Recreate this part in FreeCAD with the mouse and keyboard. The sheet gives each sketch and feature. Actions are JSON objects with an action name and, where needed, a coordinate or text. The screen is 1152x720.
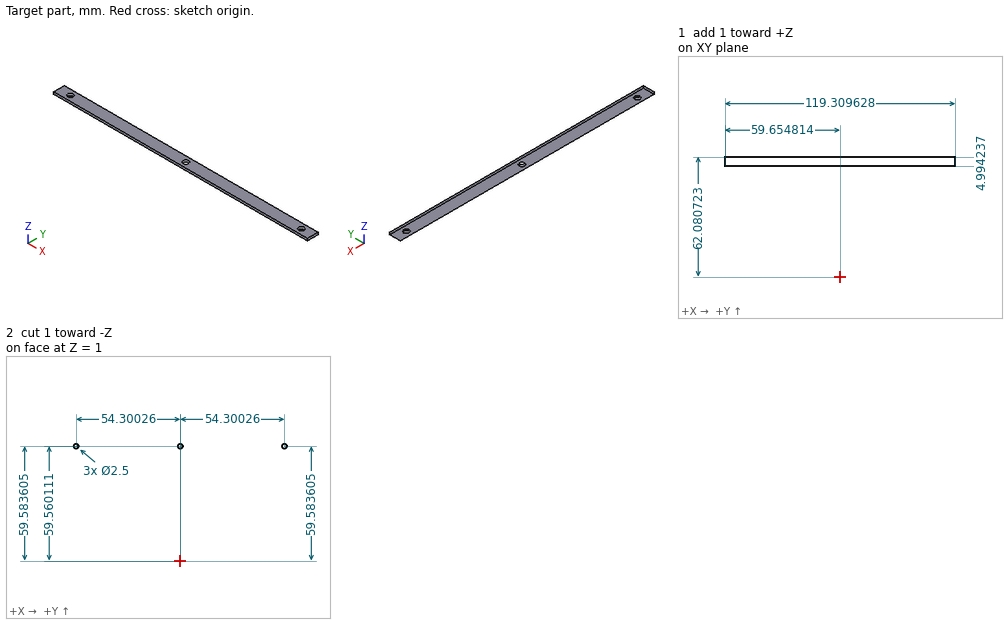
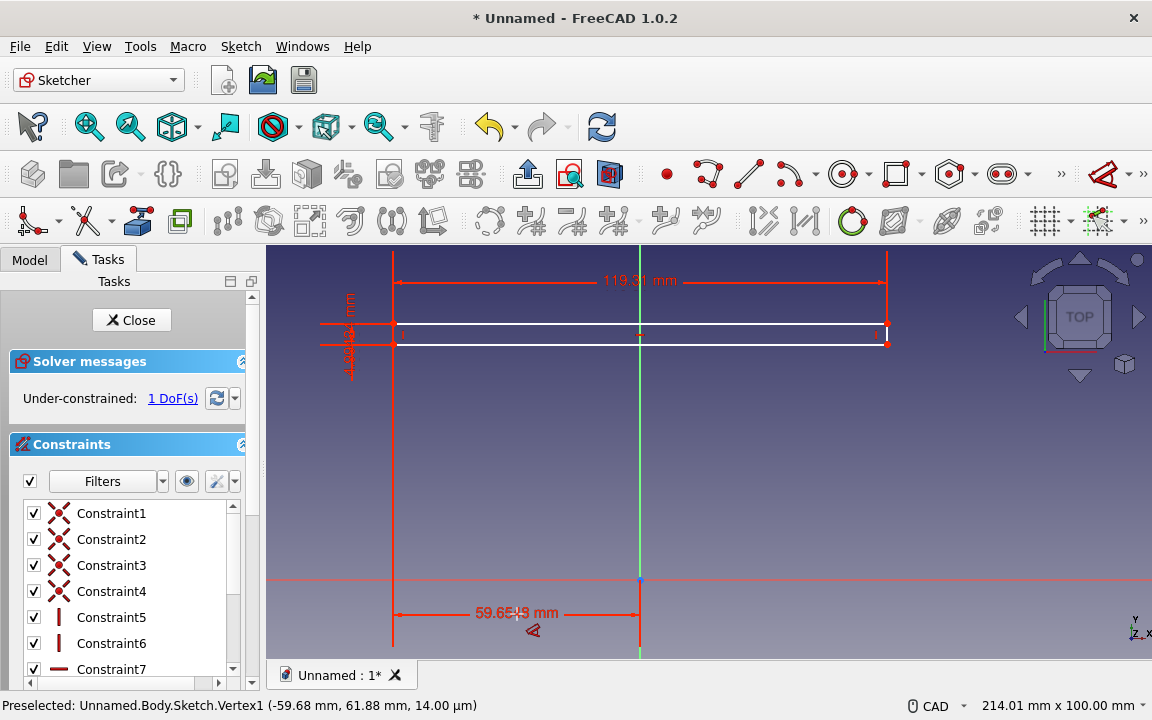
{"action": "left_click", "coordinate": [393, 324]}
{"action": "left_click", "coordinate": [359, 452]}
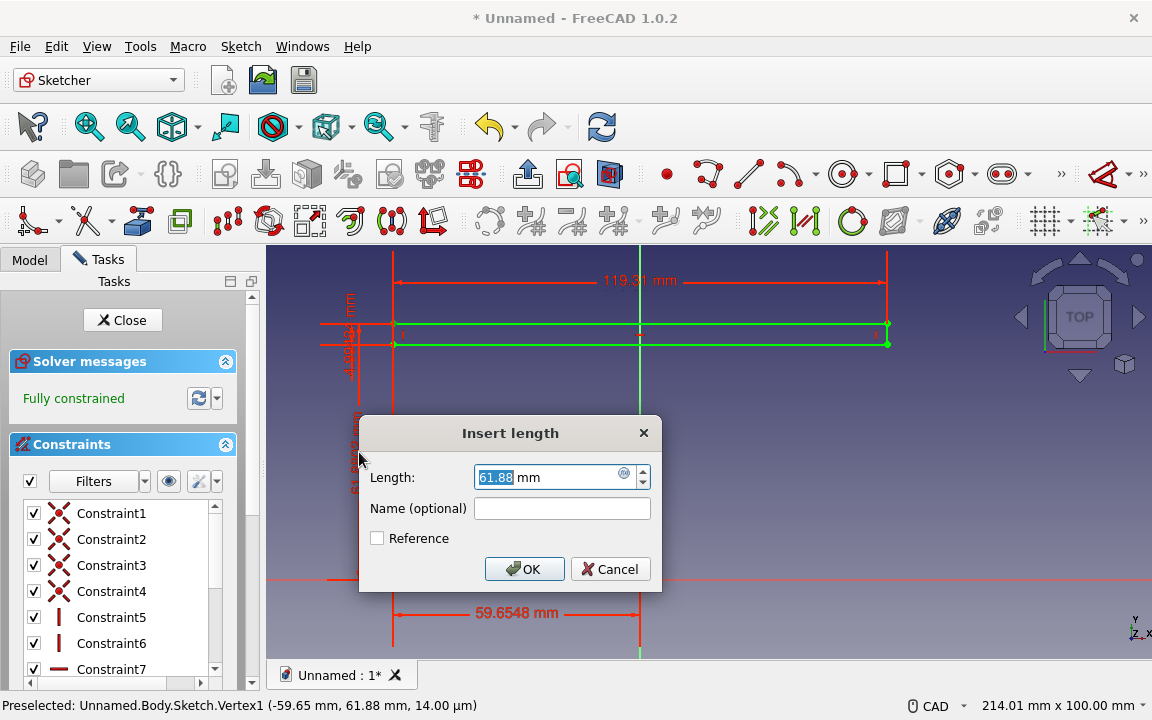
{"action": "type", "text": "62.080723"}
{"action": "key", "text": "Return"}
{"action": "key", "text": "Escape"}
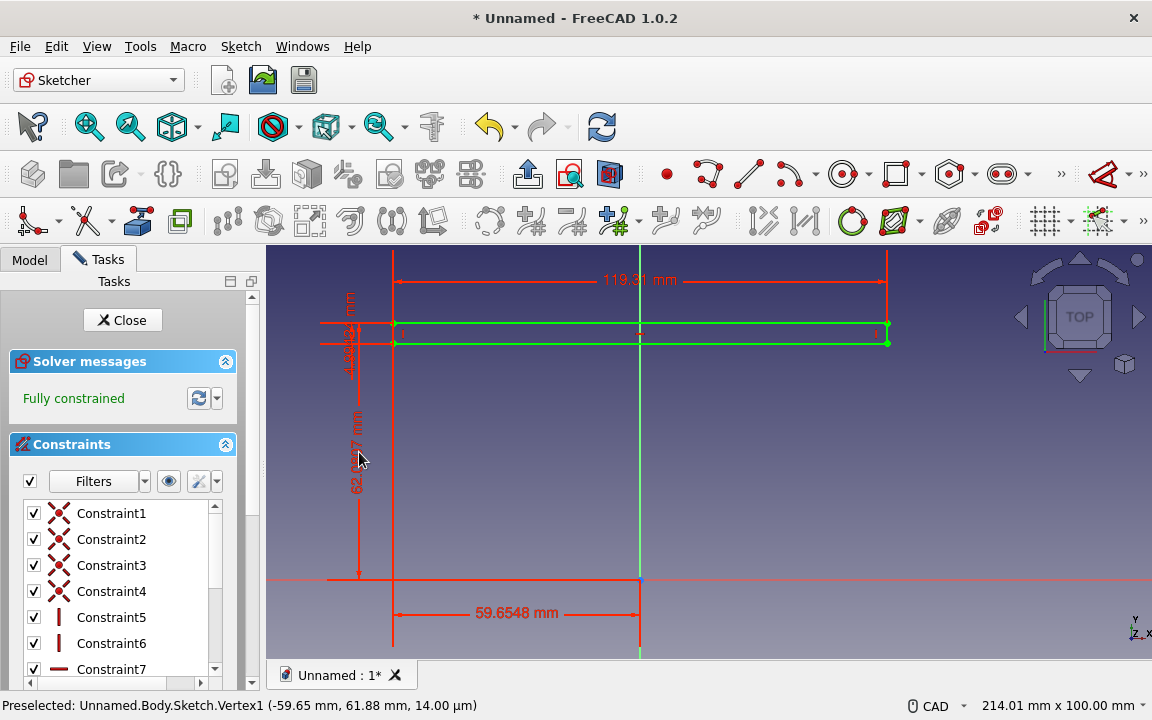
{"action": "left_click", "coordinate": [123, 320]}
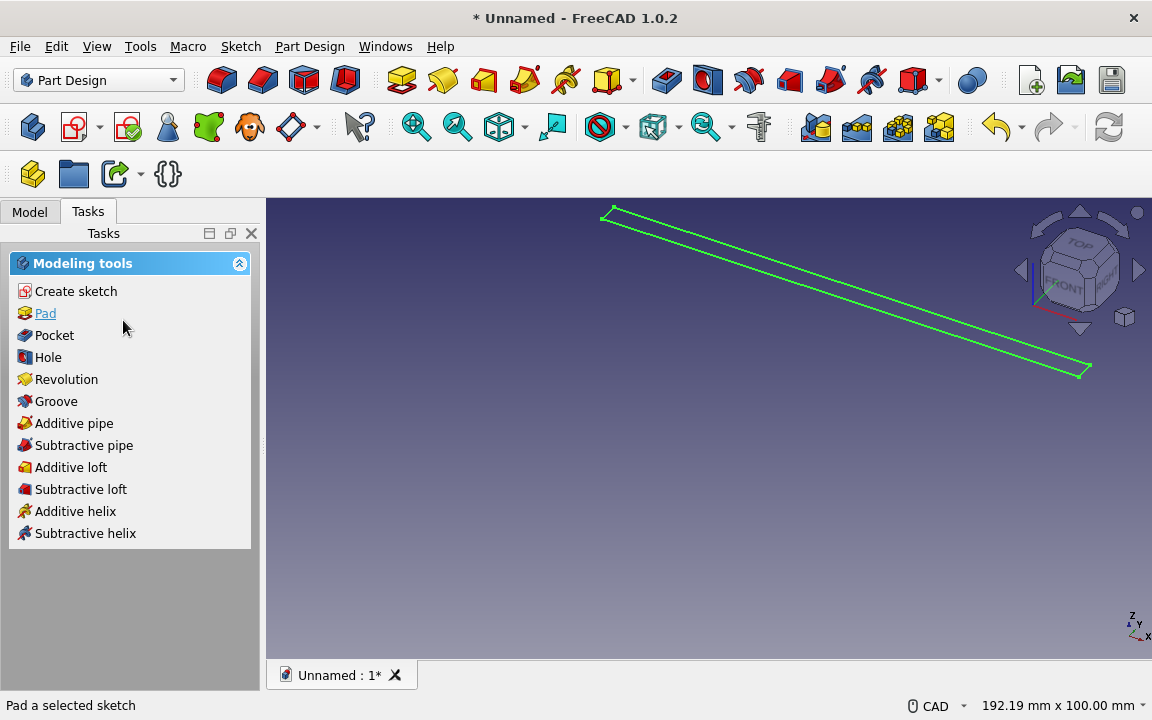
{"action": "left_click", "coordinate": [402, 80]}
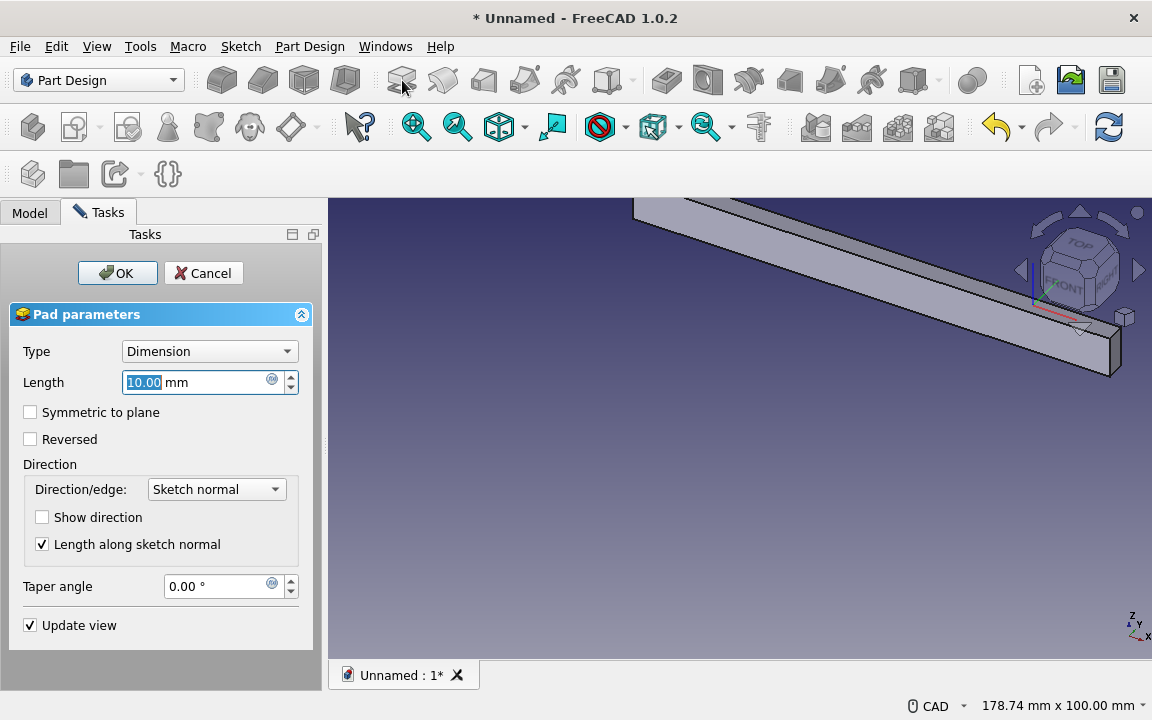
{"action": "type", "text": "1"}
{"action": "key", "text": "Tab"}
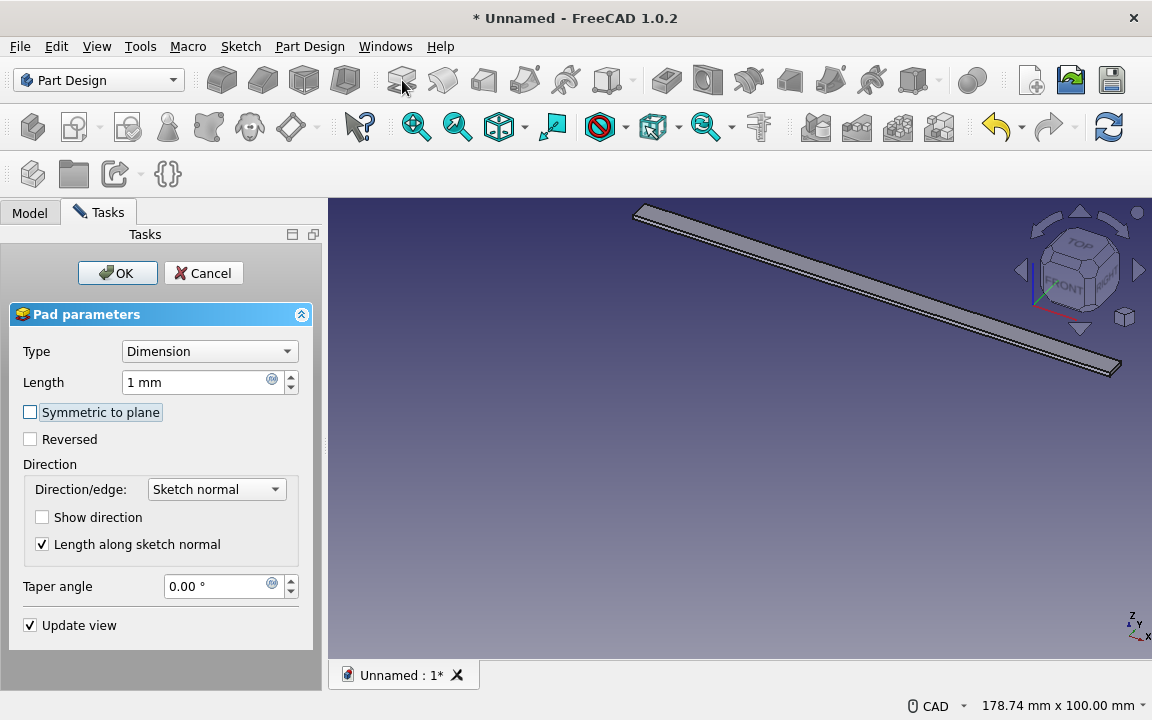
{"action": "left_click", "coordinate": [118, 273]}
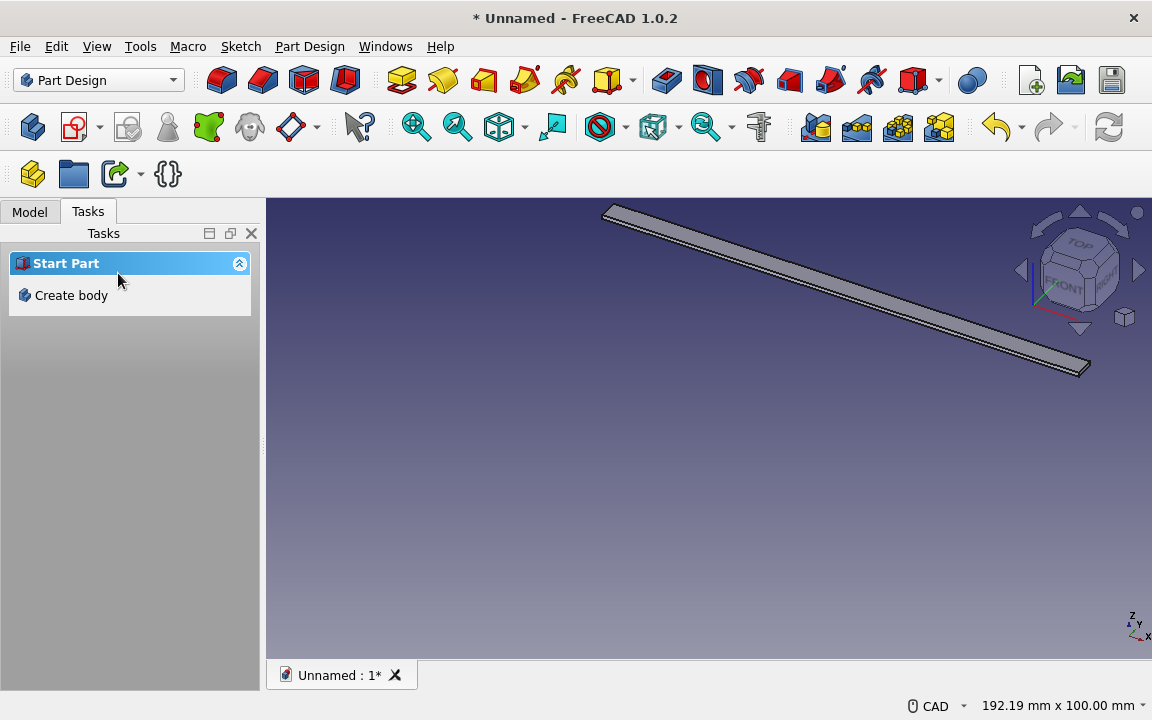
{"action": "key", "text": "0"}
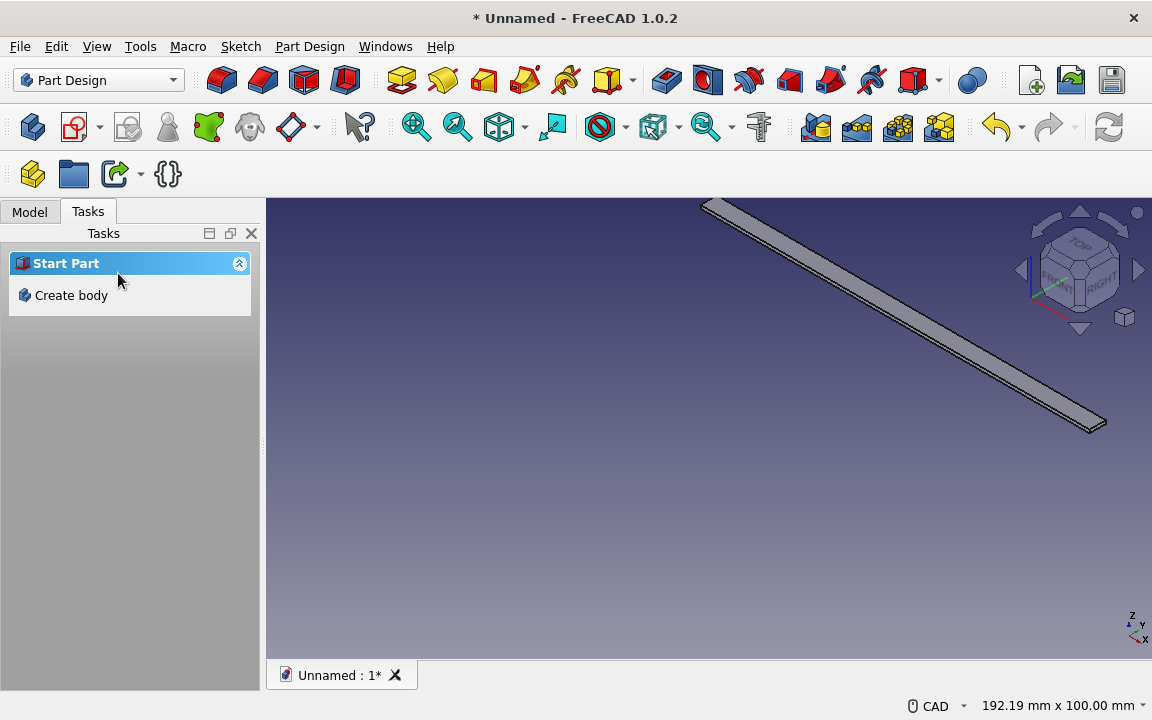
{"action": "key", "text": "v f"}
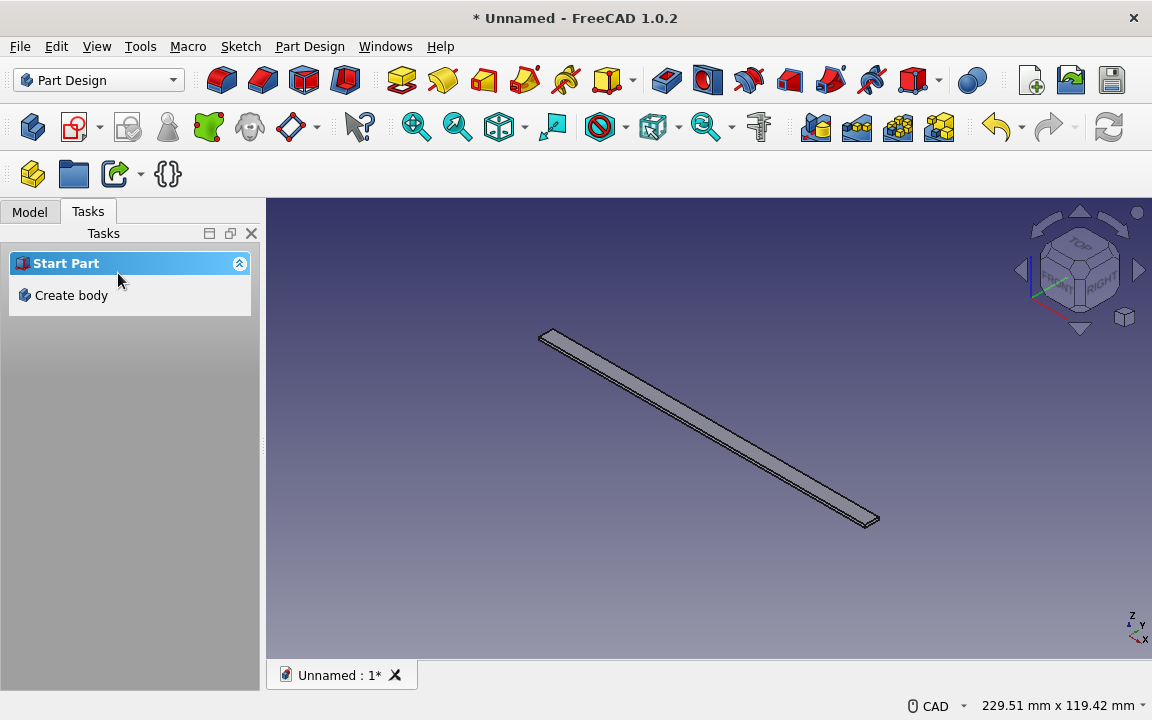
{"action": "left_click", "coordinate": [851, 505]}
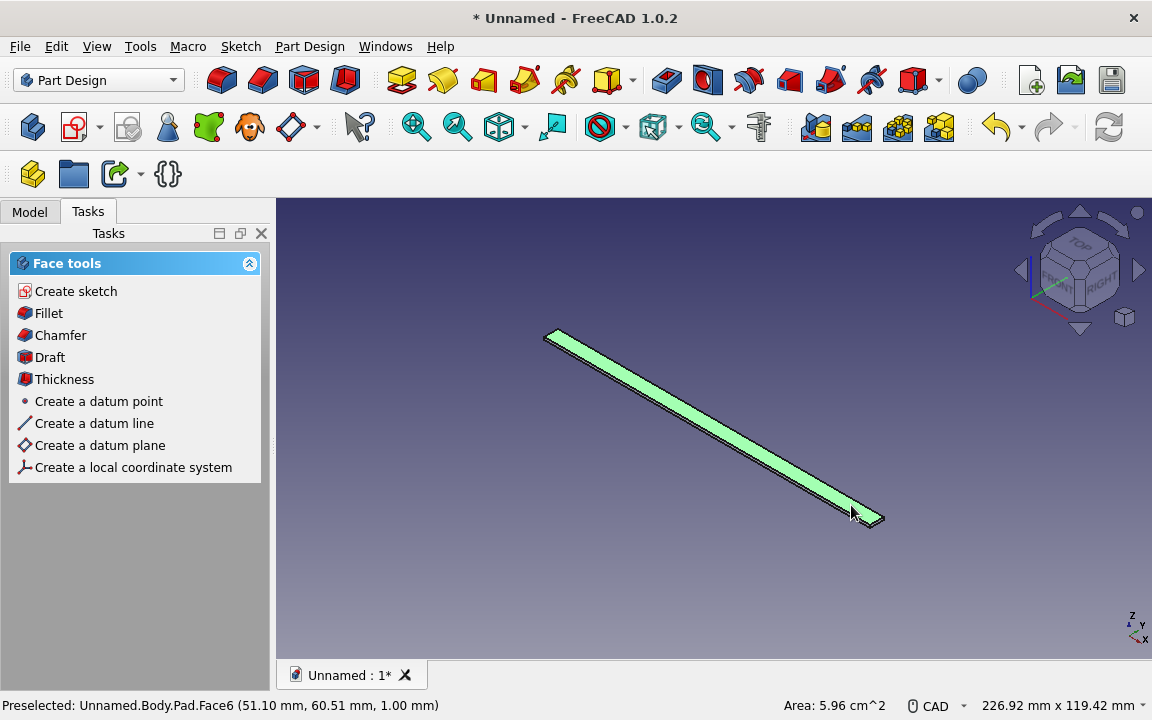
{"action": "left_click", "coordinate": [74, 128]}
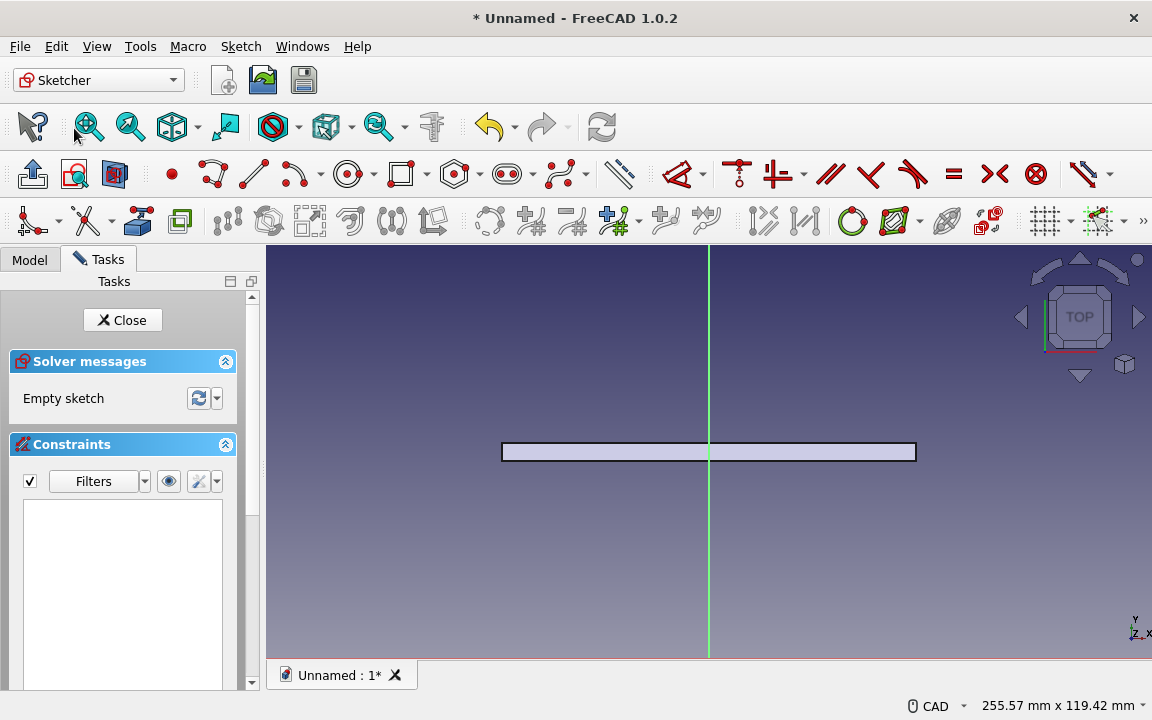
{"action": "scroll", "coordinate": [331, 273], "scroll_direction": "down", "scroll_amount": 1}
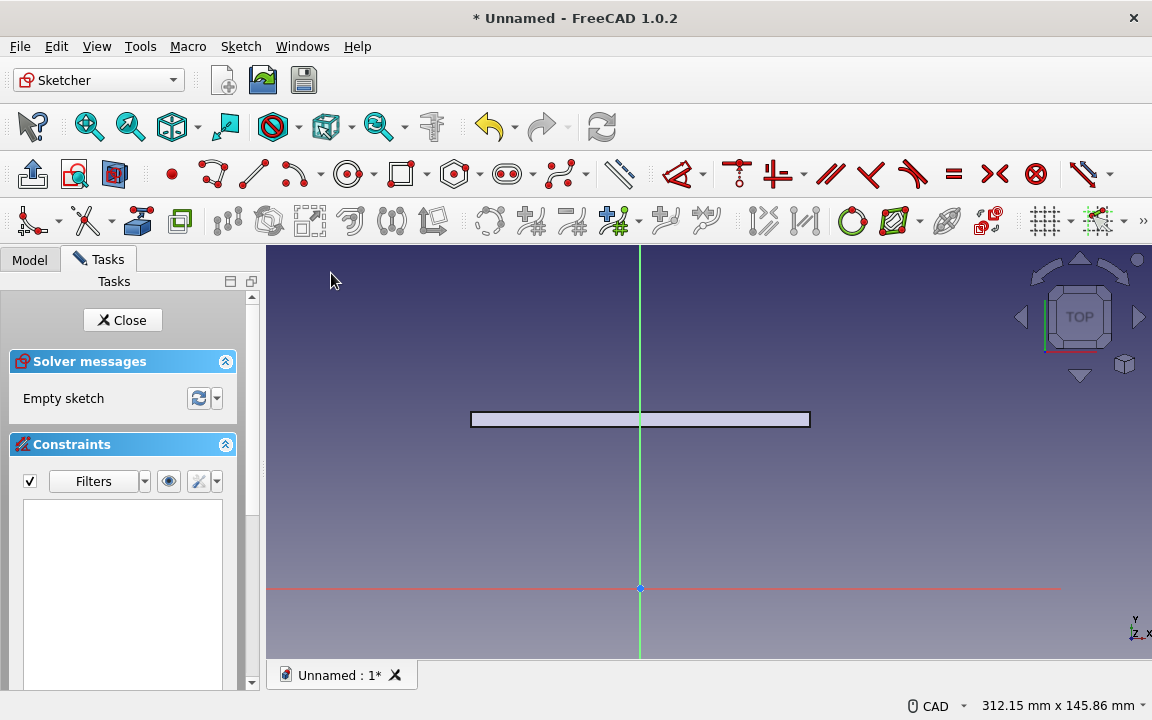
{"action": "scroll", "coordinate": [640, 605], "scroll_direction": "up", "scroll_amount": 2}